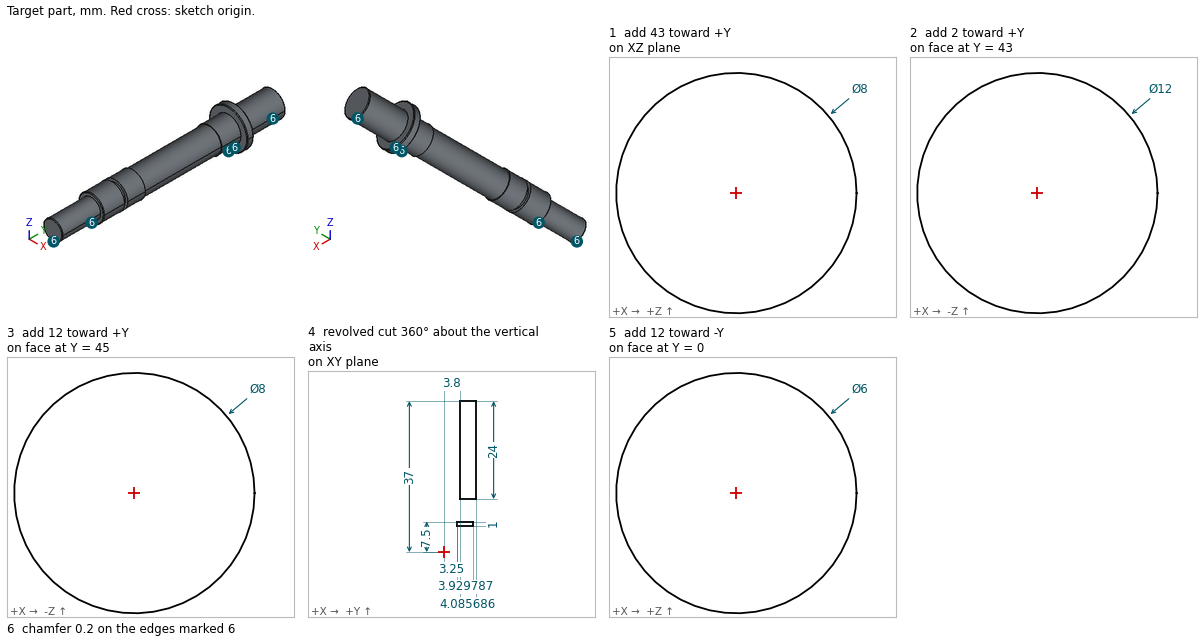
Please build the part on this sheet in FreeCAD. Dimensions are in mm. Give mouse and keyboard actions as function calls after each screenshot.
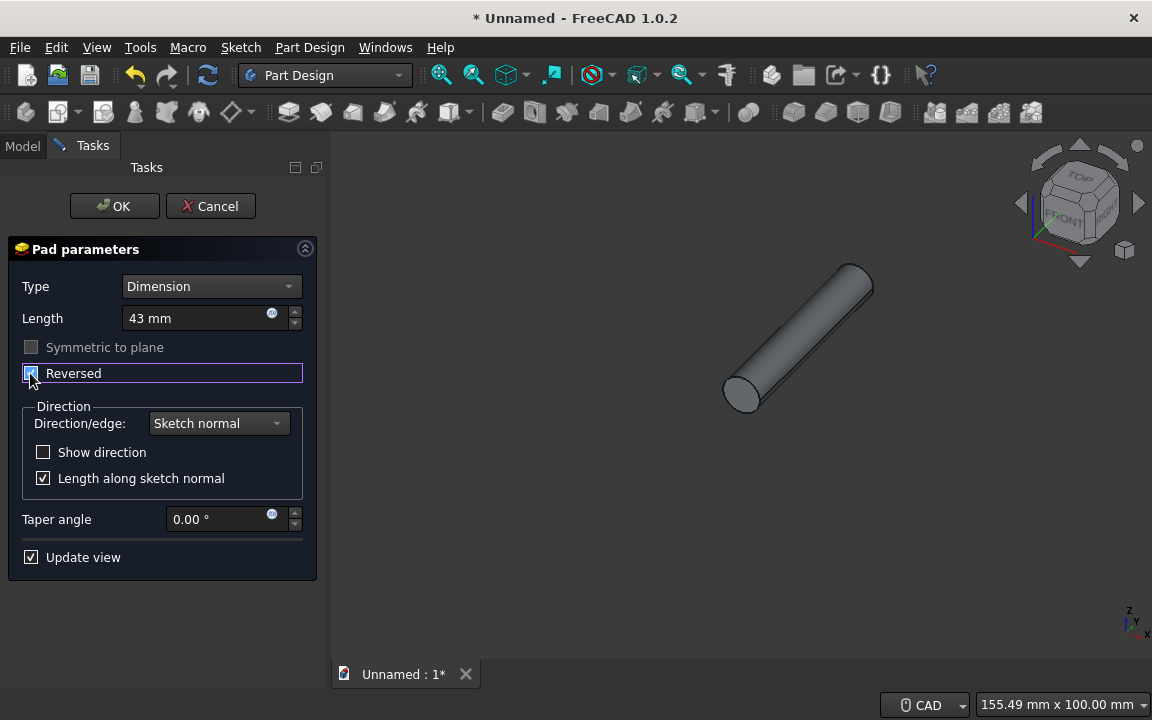
click(115, 206)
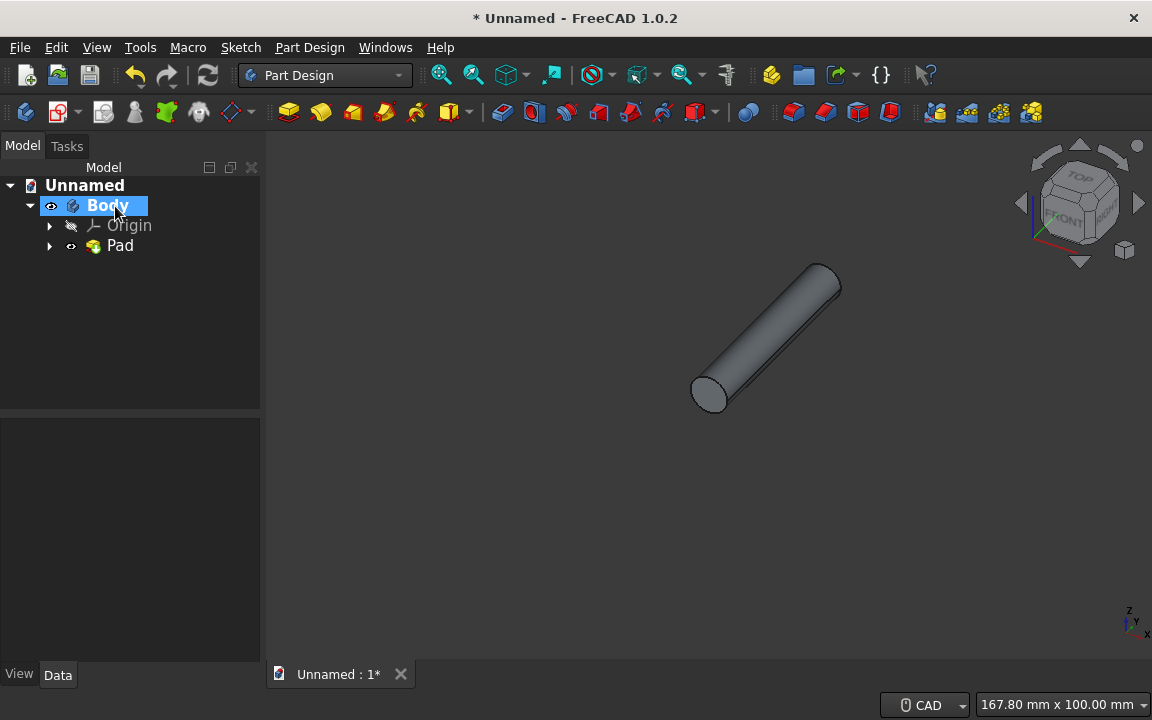
click(442, 76)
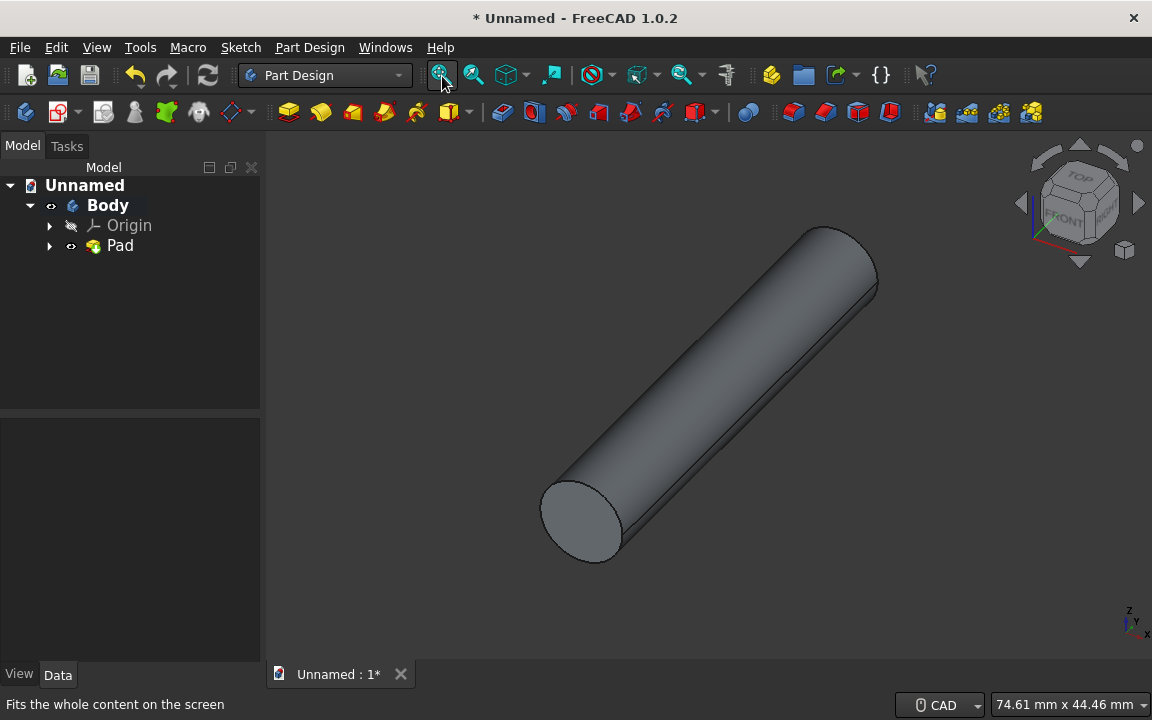
key(4)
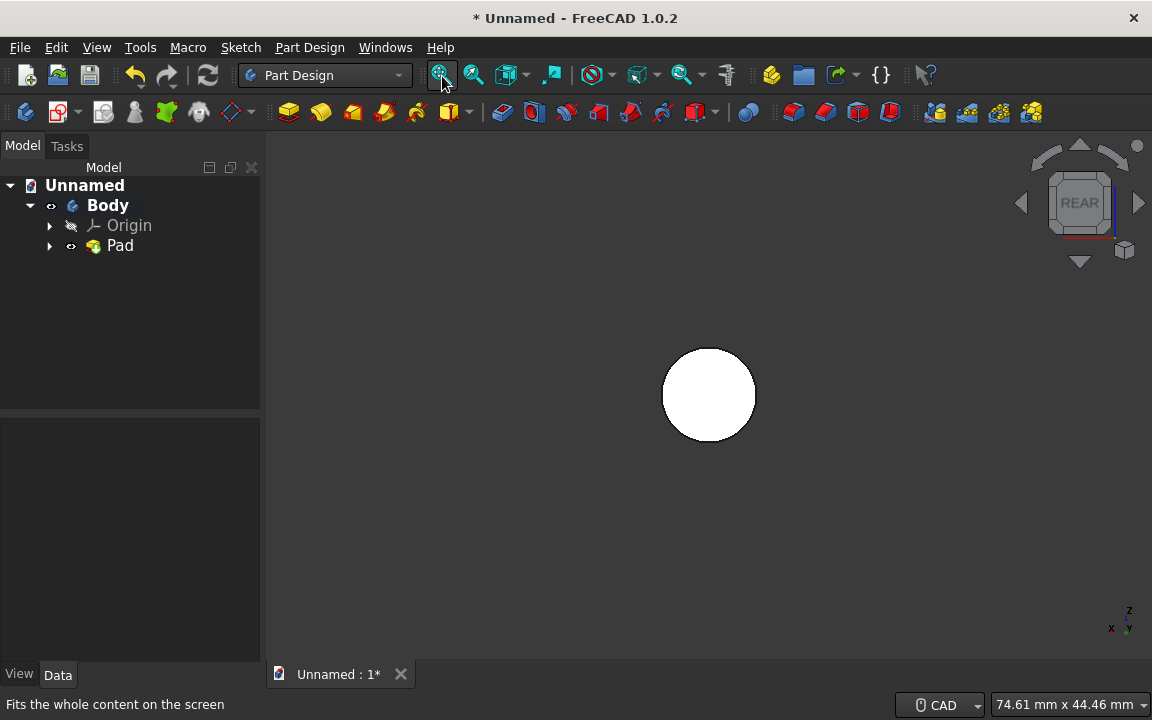
click(442, 76)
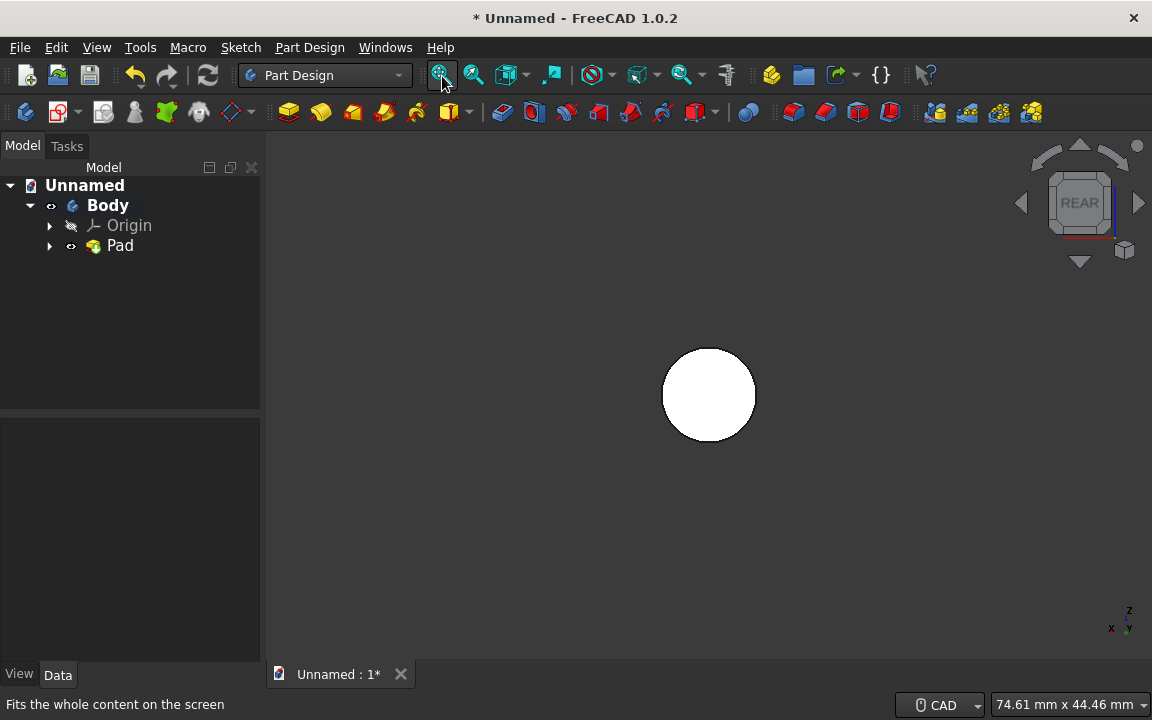
click(709, 394)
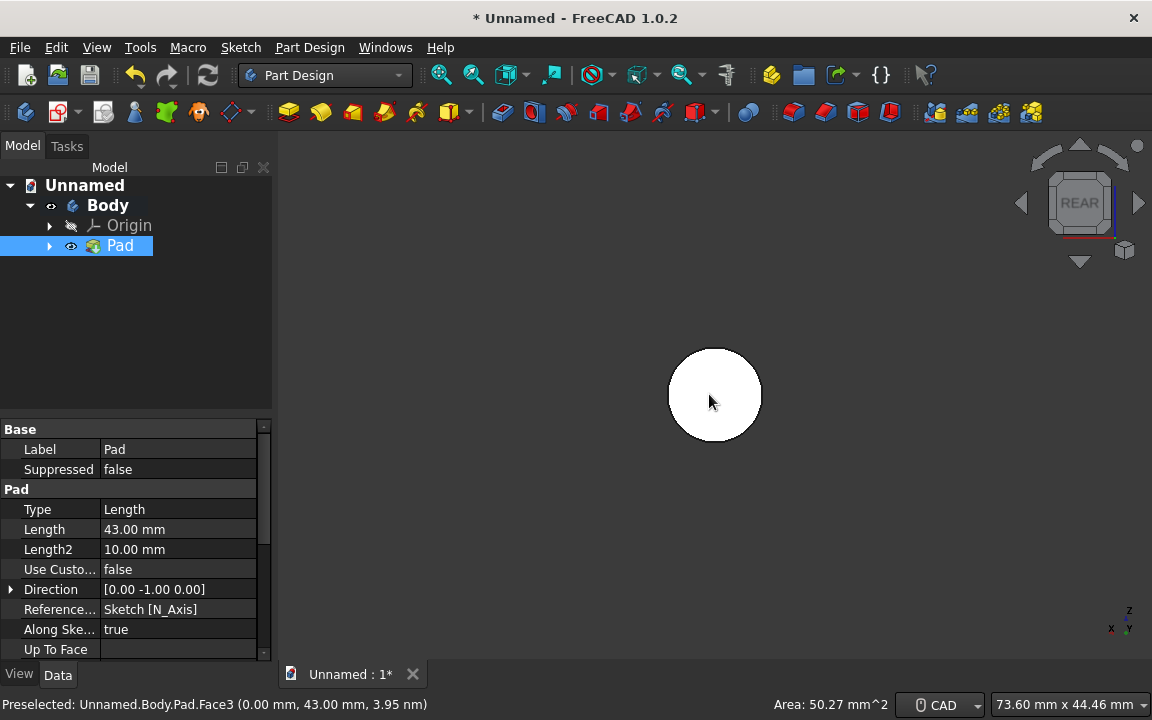
click(58, 112)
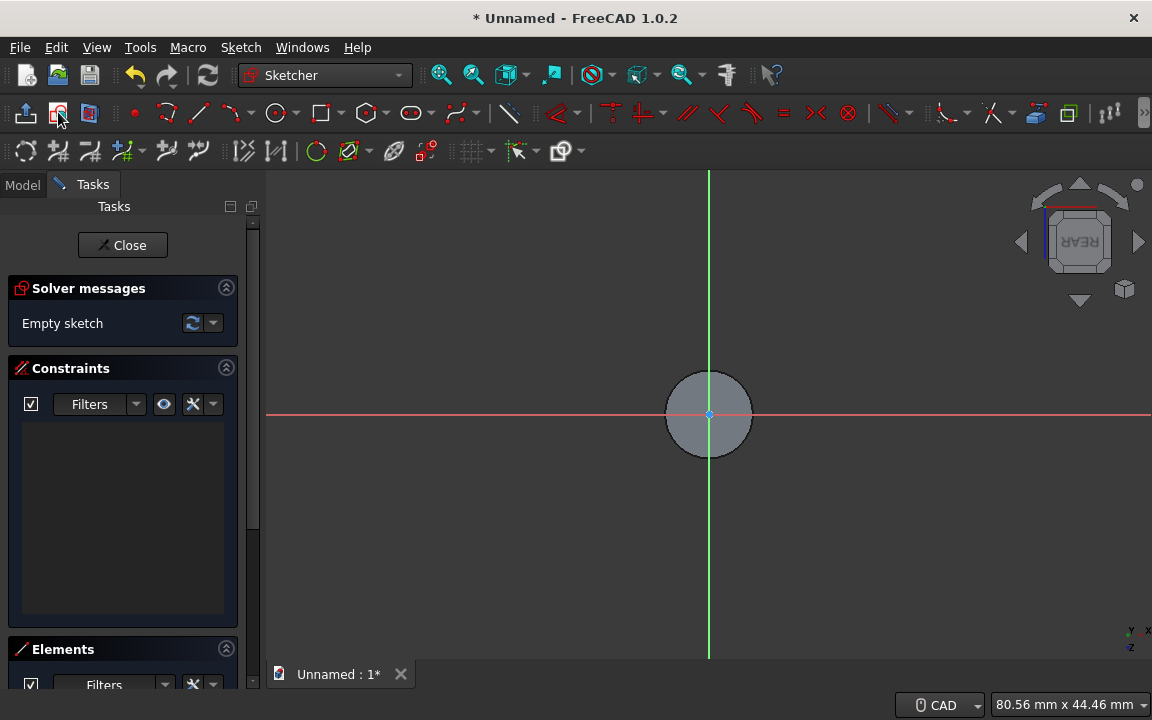
scroll(765, 414, up, 4)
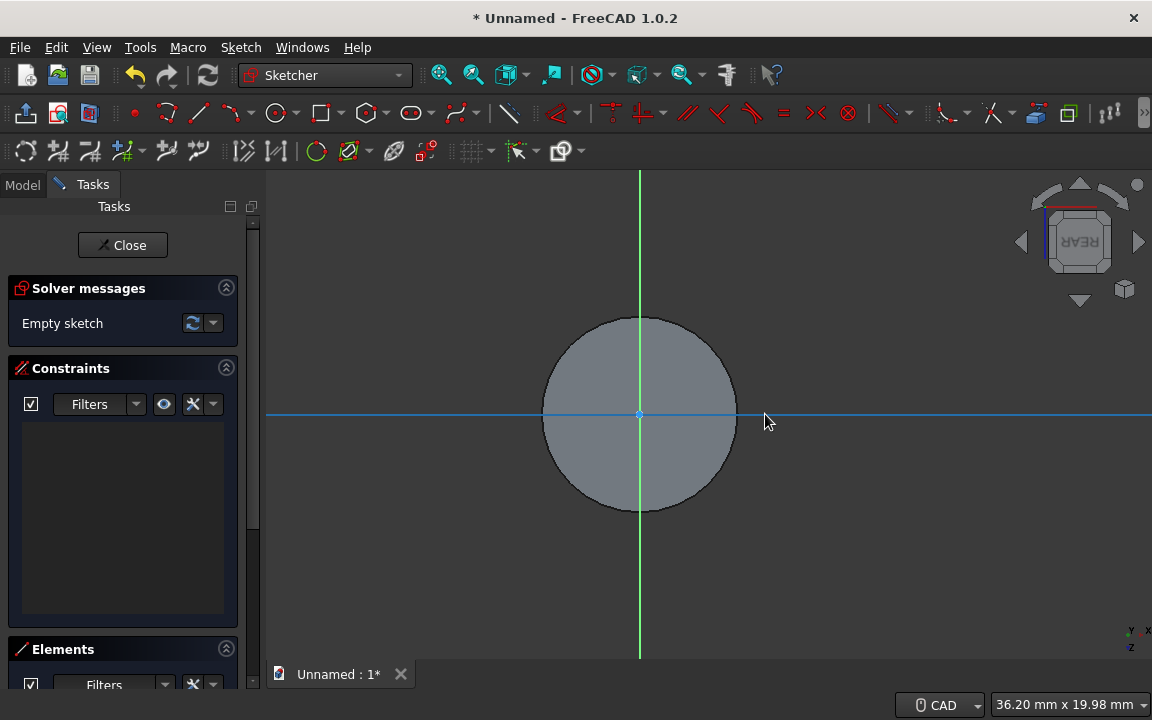
click(276, 114)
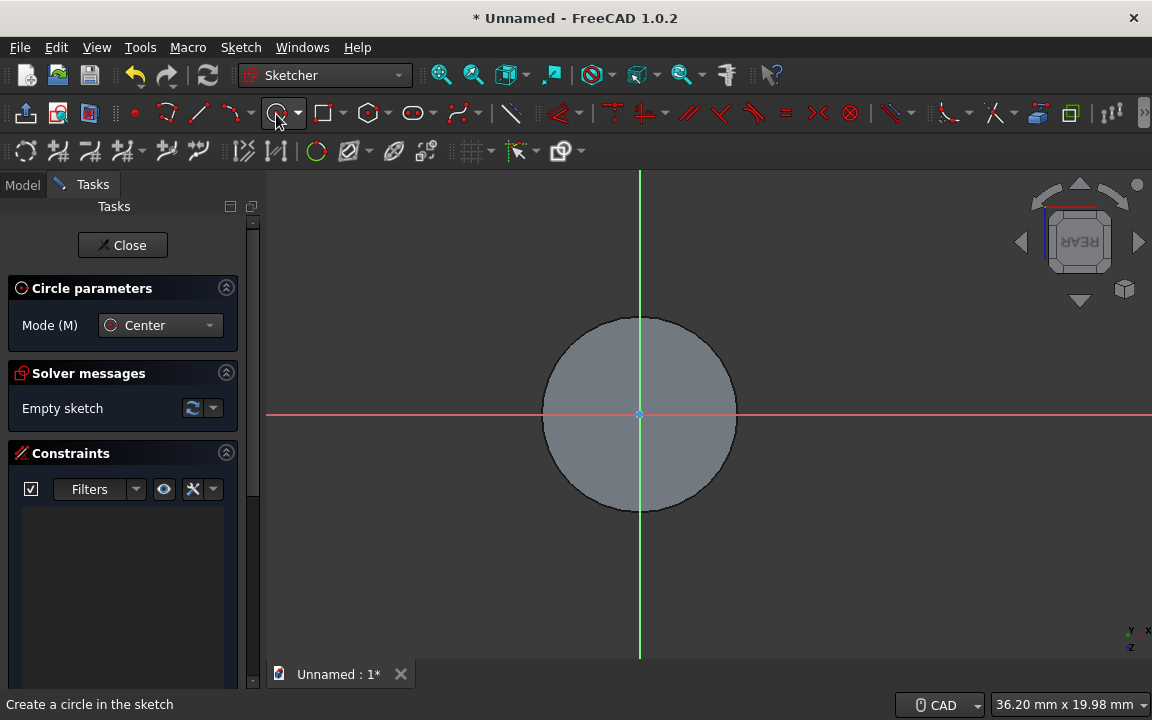
click(640, 414)
move(744, 311)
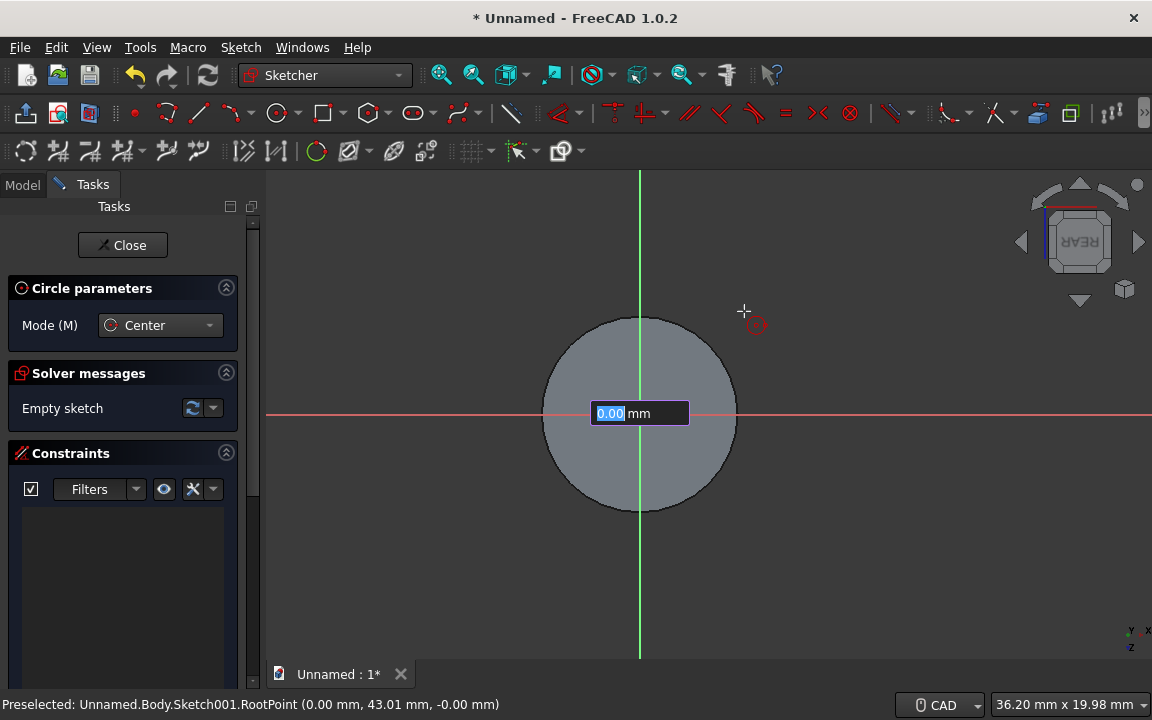
text(12)
key(Return)
key(Escape)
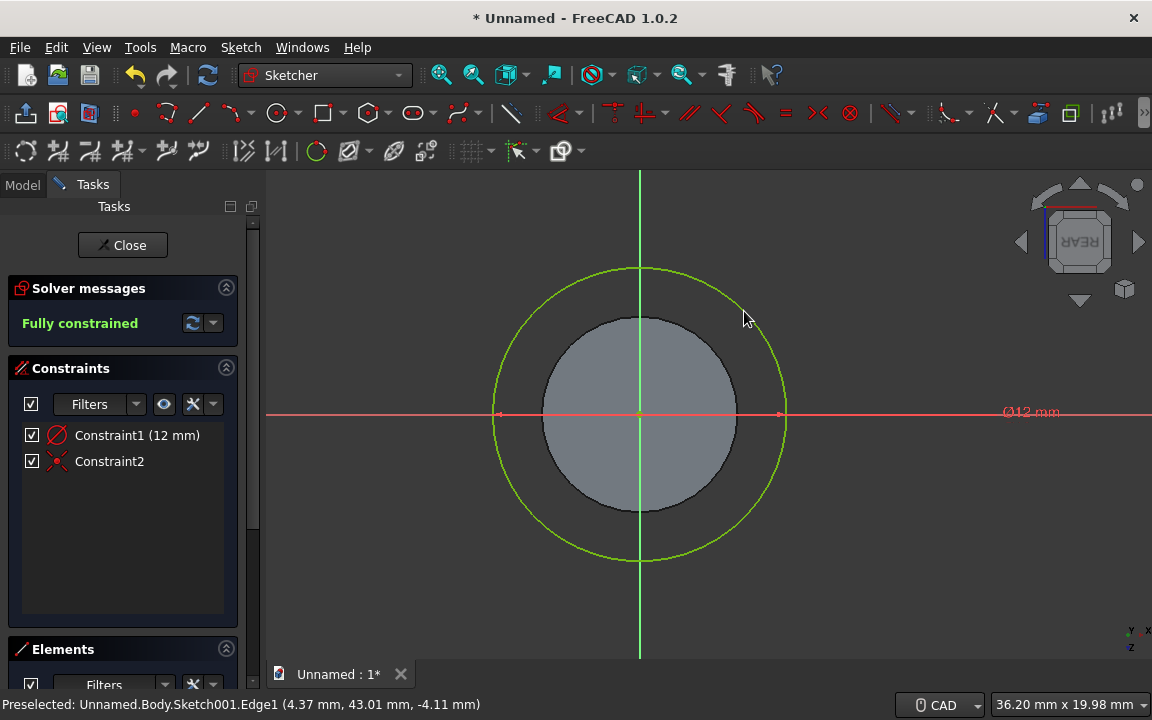
click(123, 245)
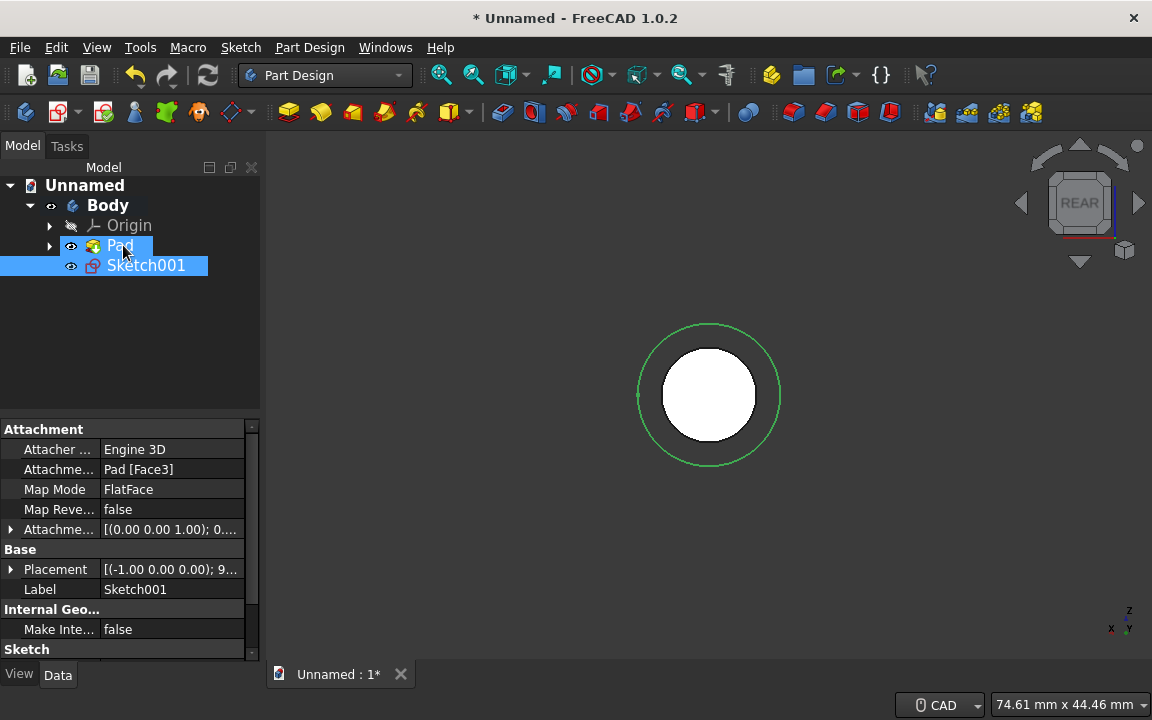
click(290, 112)